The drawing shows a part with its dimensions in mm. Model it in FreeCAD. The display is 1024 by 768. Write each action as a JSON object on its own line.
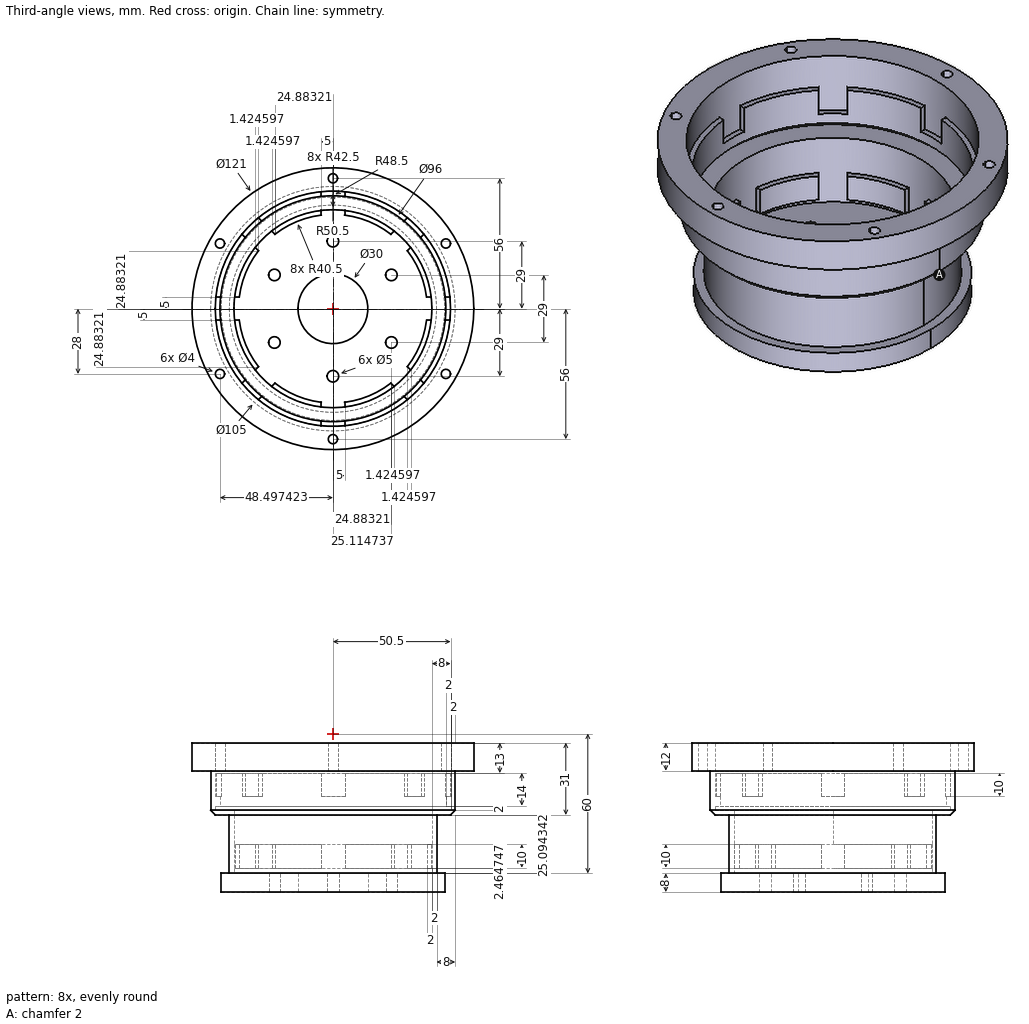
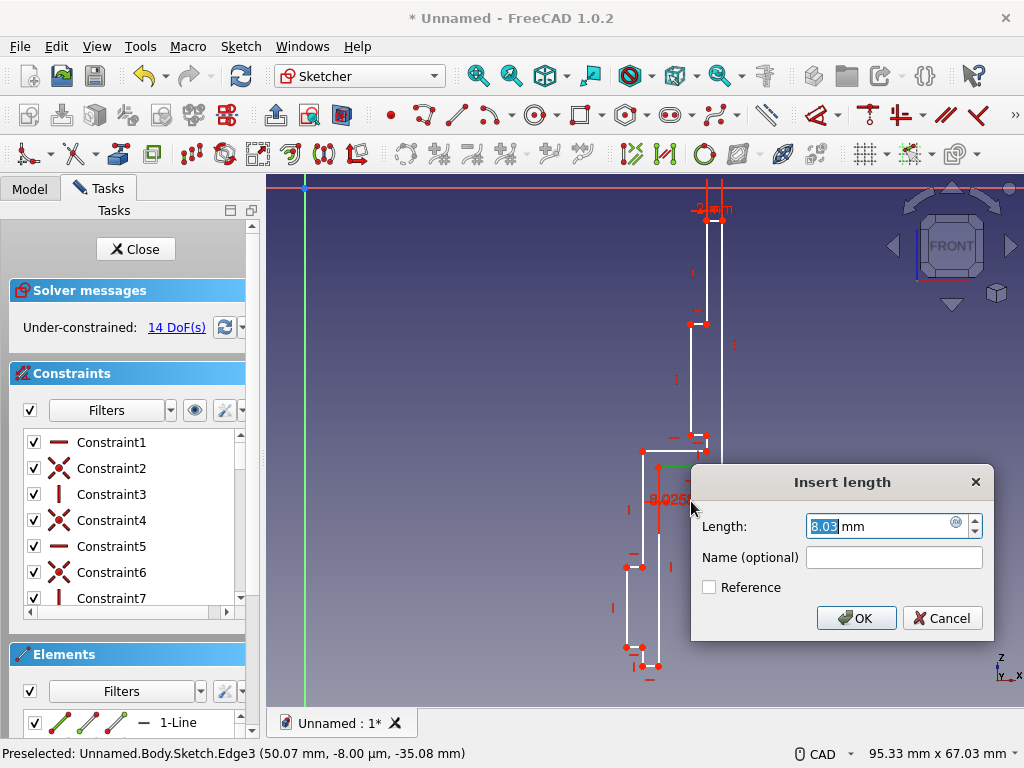
{"action": "type", "text": "8"}
{"action": "key", "text": "Return"}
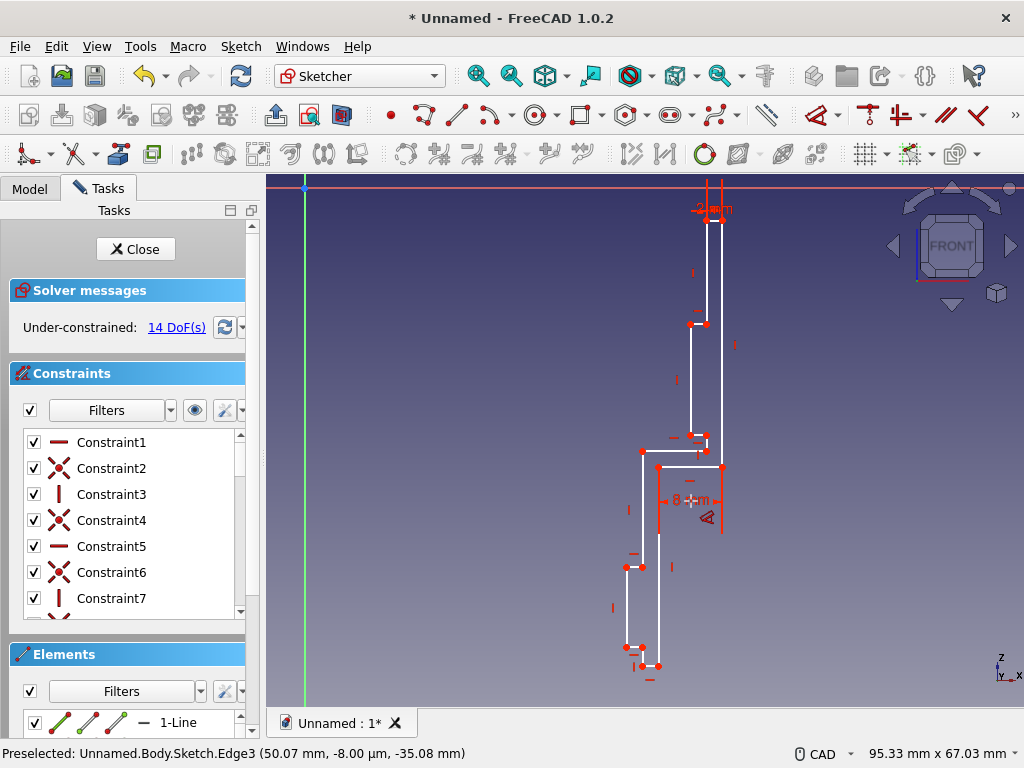
{"action": "scroll", "coordinate": [651, 666], "scroll_direction": "up", "scroll_amount": 5}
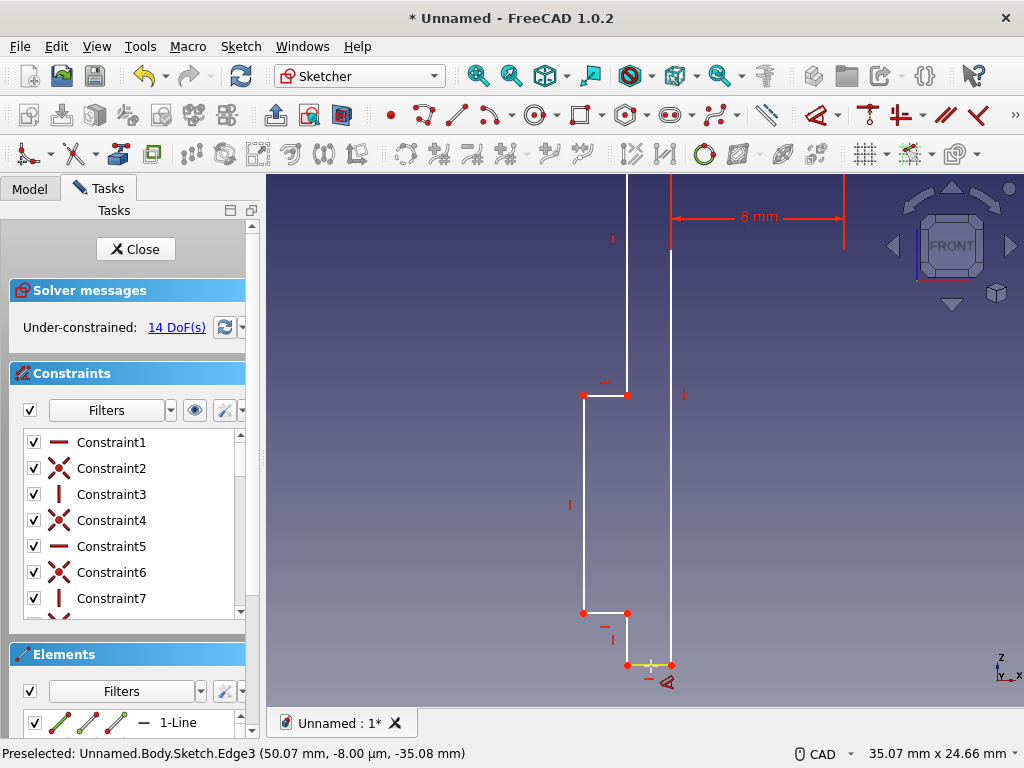
{"action": "left_click", "coordinate": [649, 665]}
{"action": "left_click", "coordinate": [649, 631]}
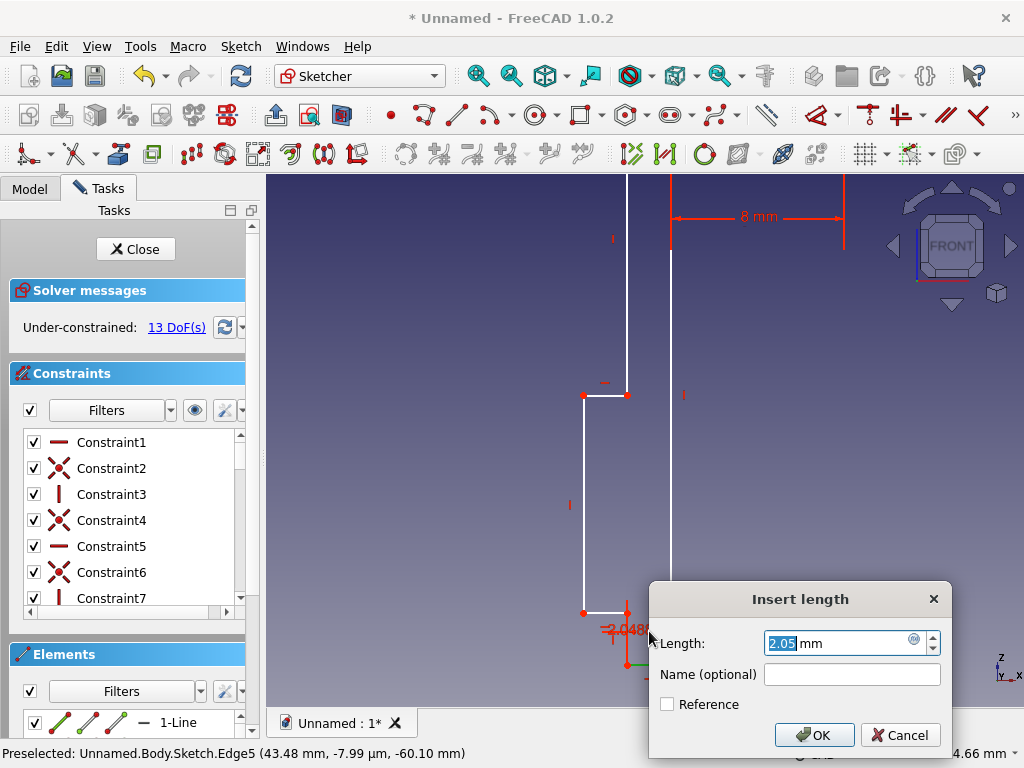
{"action": "type", "text": "2"}
{"action": "key", "text": "Return"}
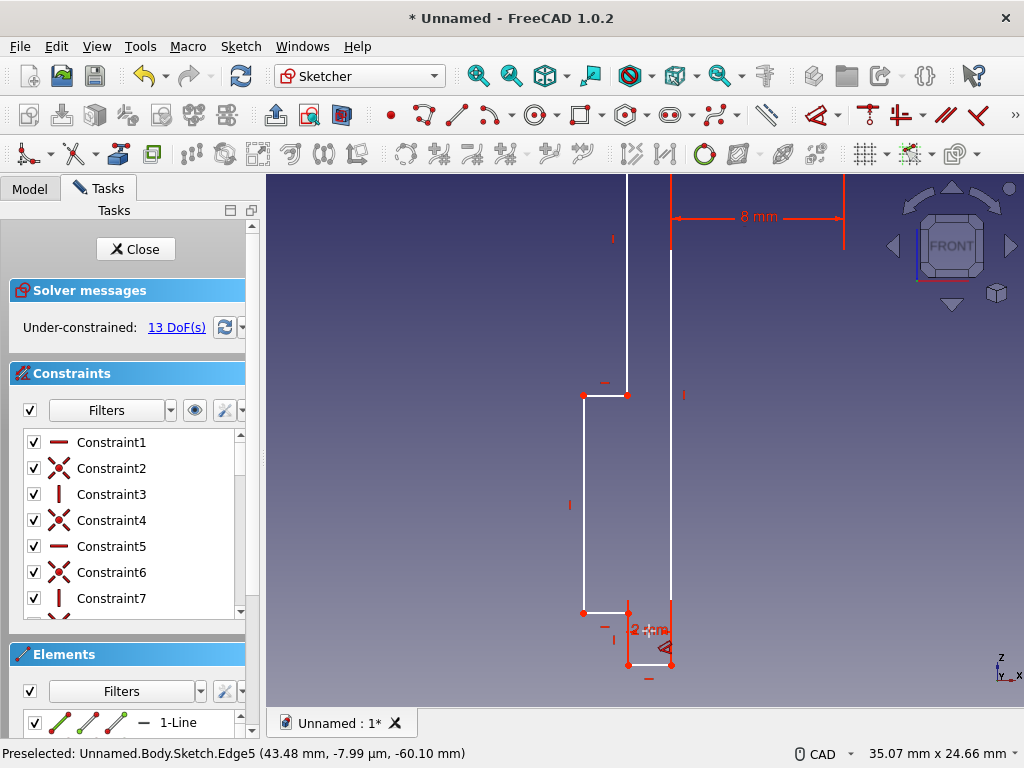
{"action": "left_click", "coordinate": [615, 613]}
{"action": "left_click", "coordinate": [606, 579]}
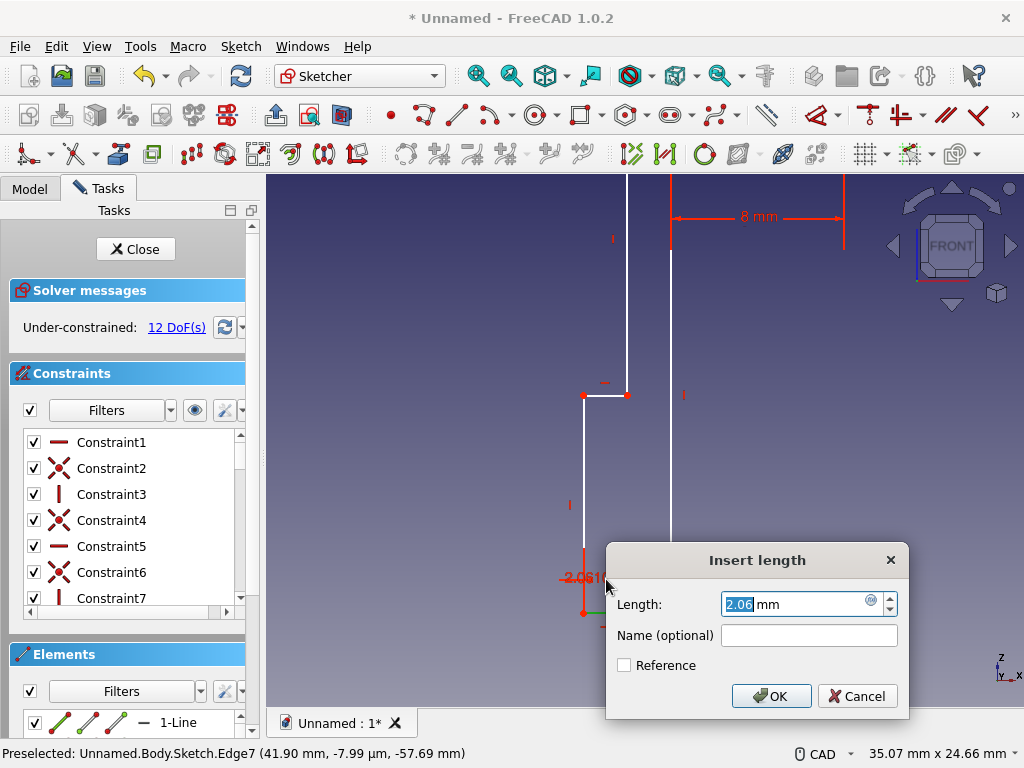
{"action": "type", "text": "2"}
{"action": "key", "text": "Return"}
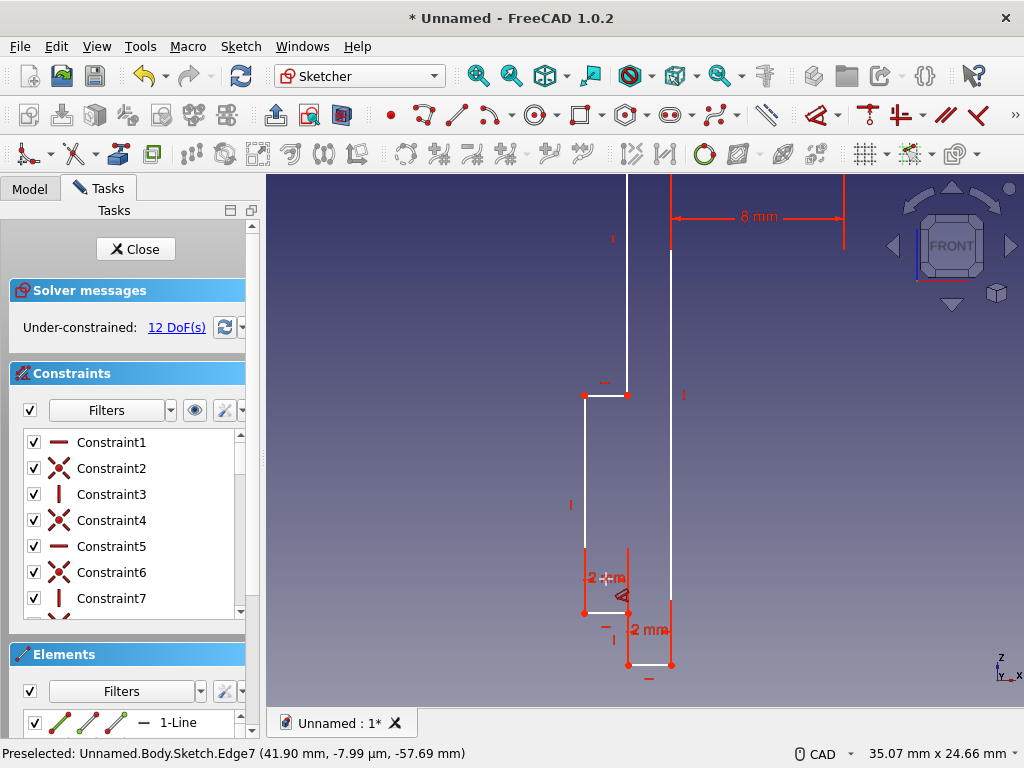
{"action": "left_click", "coordinate": [598, 396]}
{"action": "left_click", "coordinate": [606, 430]}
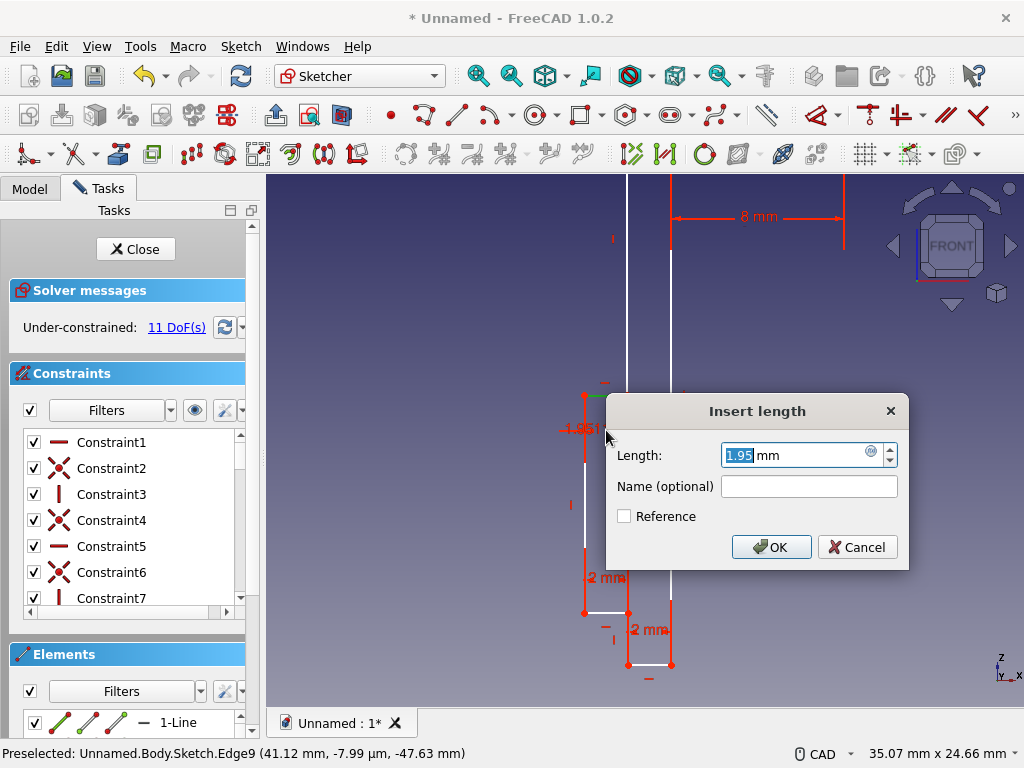
{"action": "type", "text": "2"}
{"action": "key", "text": "Return"}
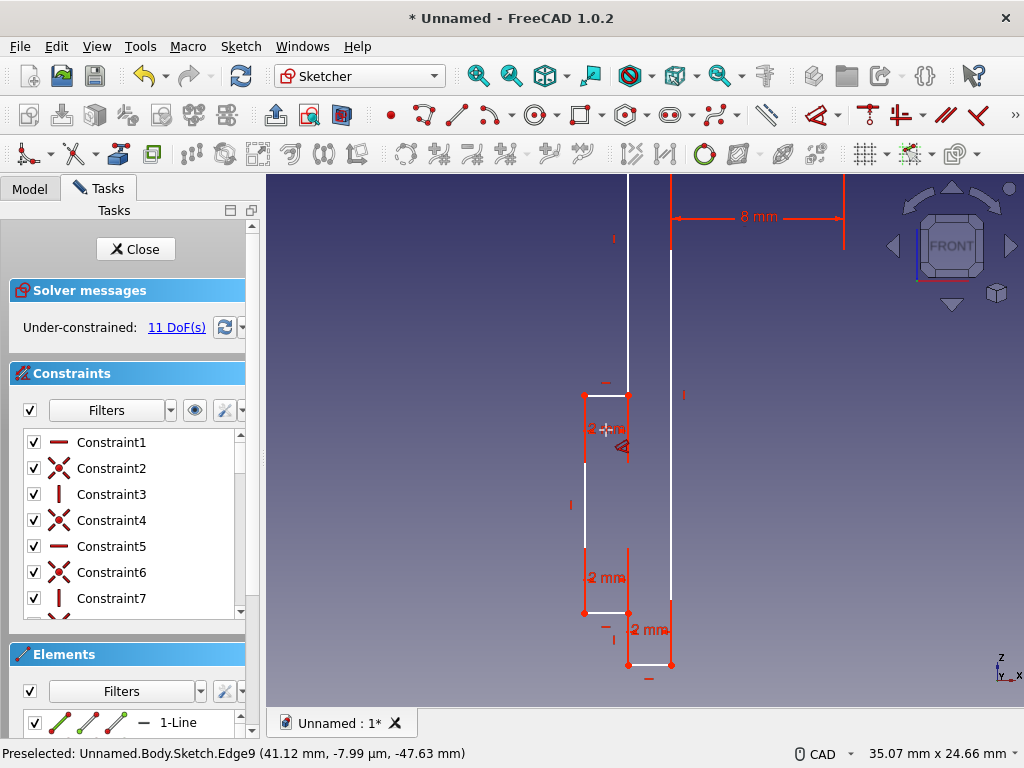
{"action": "scroll", "coordinate": [675, 580], "scroll_direction": "down", "scroll_amount": 7}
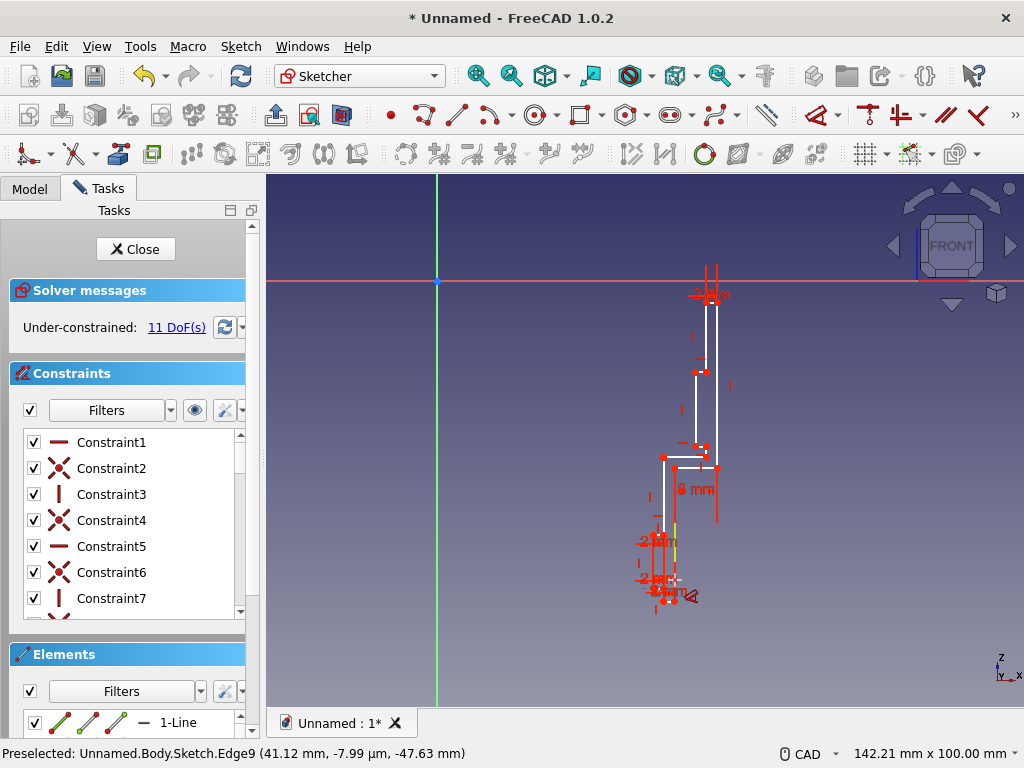
{"action": "scroll", "coordinate": [677, 457], "scroll_direction": "up", "scroll_amount": 2}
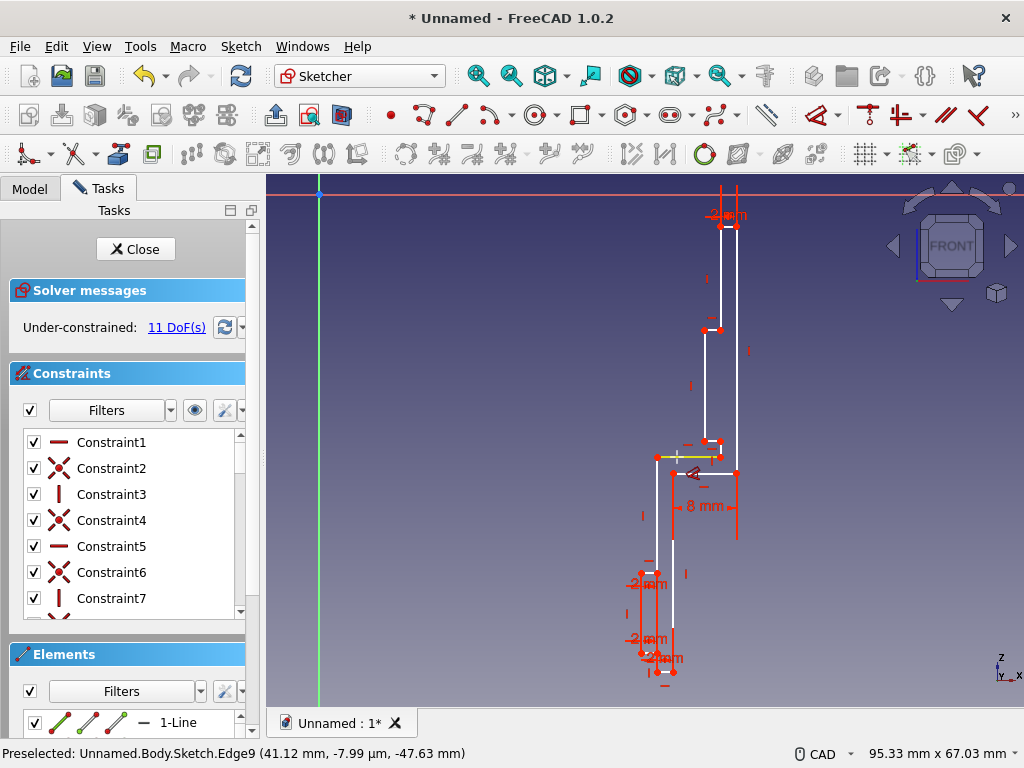
{"action": "left_click", "coordinate": [676, 457]}
{"action": "left_click", "coordinate": [689, 423]}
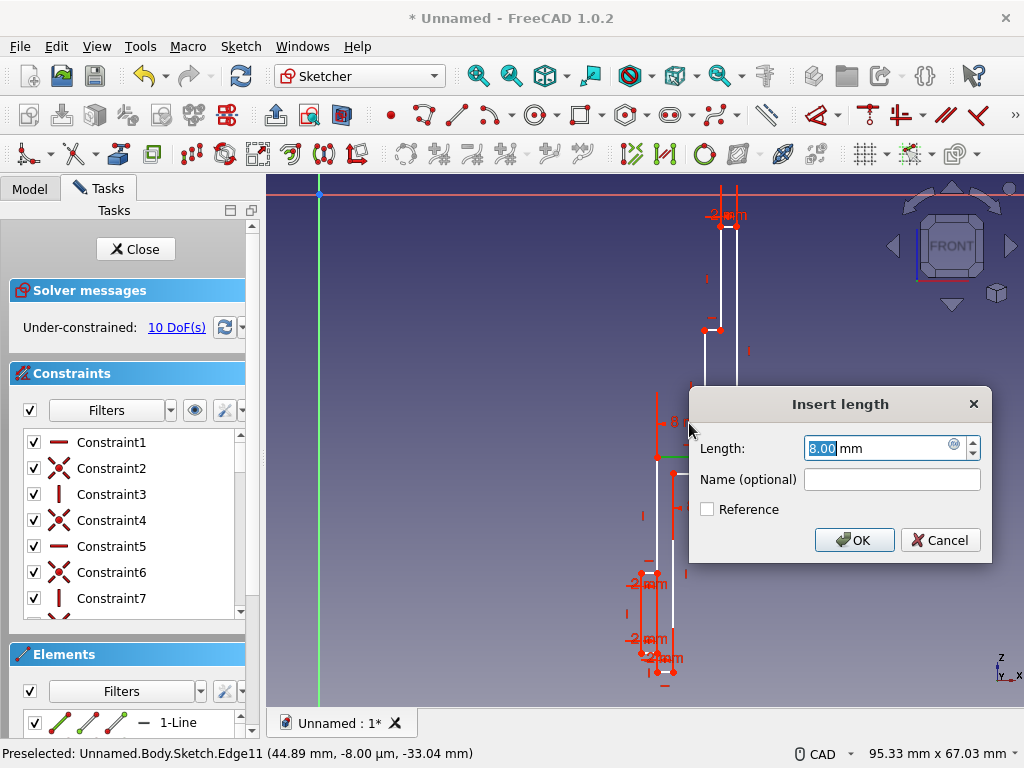
{"action": "type", "text": "8"}
{"action": "key", "text": "Return"}